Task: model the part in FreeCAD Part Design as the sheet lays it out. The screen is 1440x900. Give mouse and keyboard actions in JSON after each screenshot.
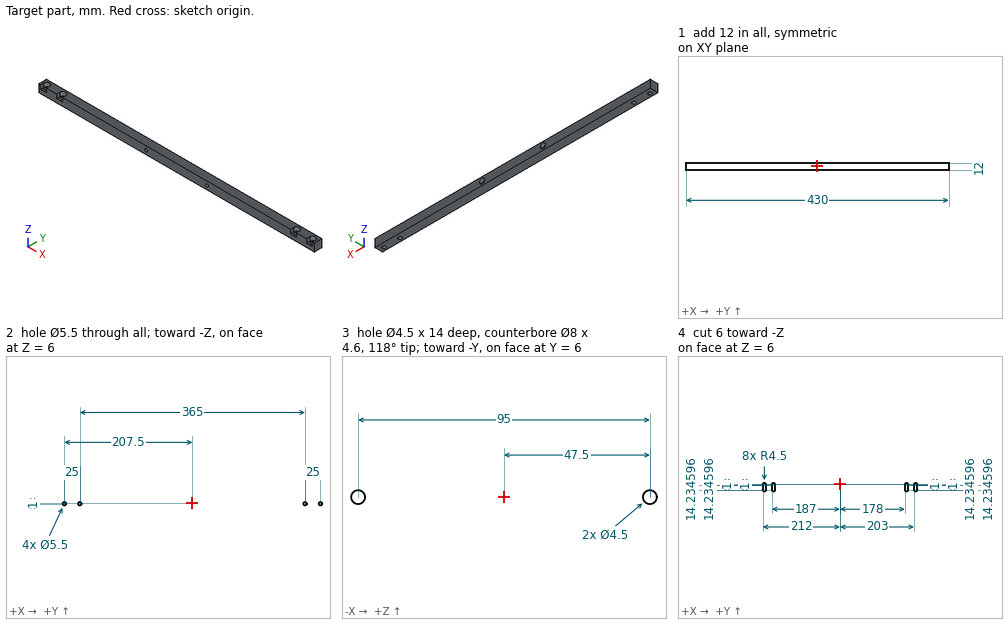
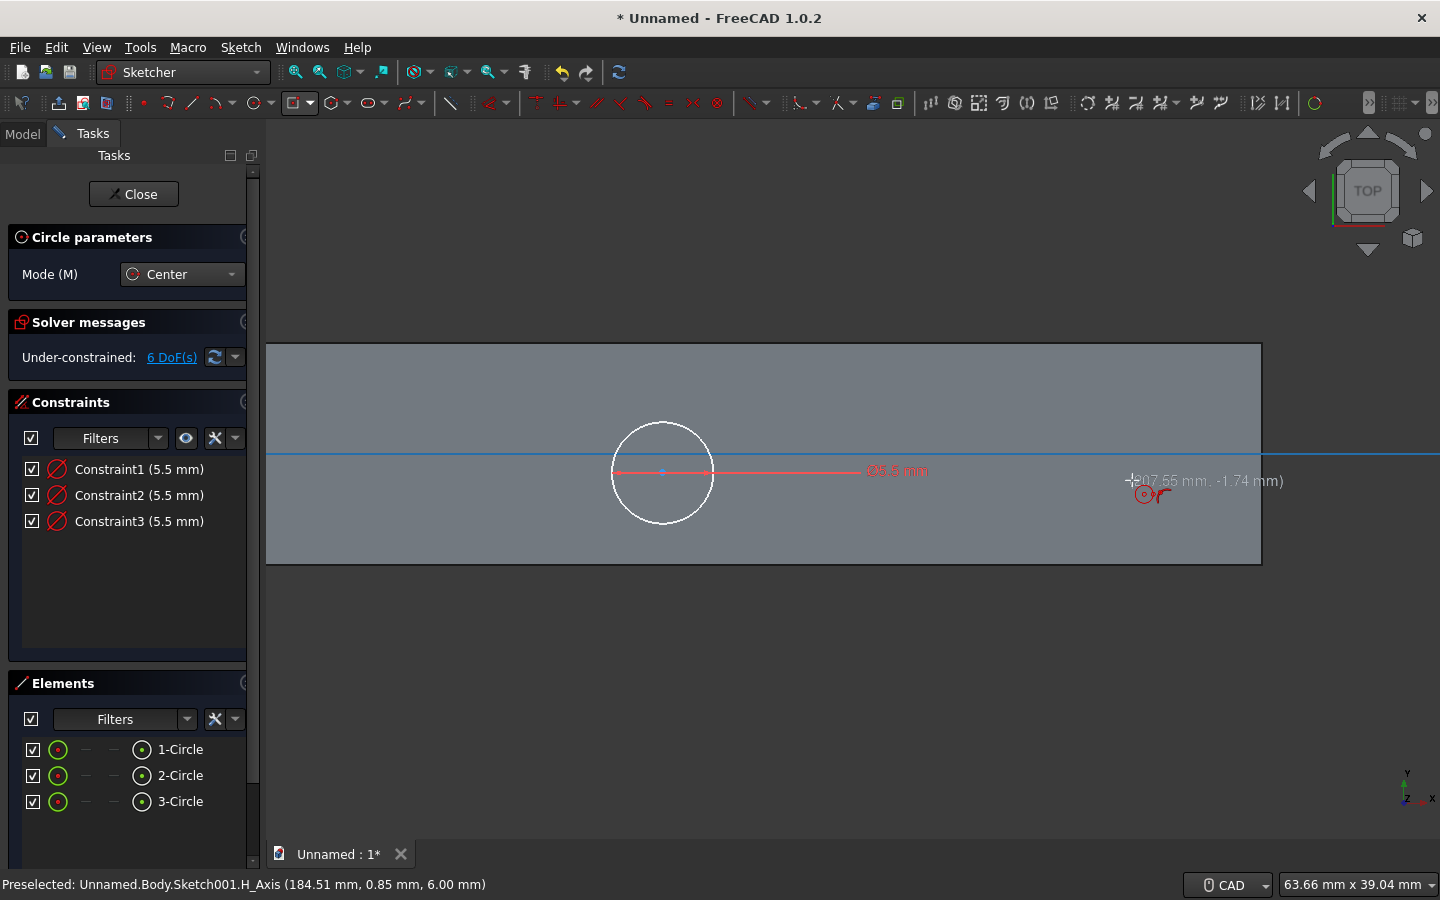
{"action": "left_click", "coordinate": [1124, 472]}
{"action": "mouse_move", "coordinate": [1160, 436]}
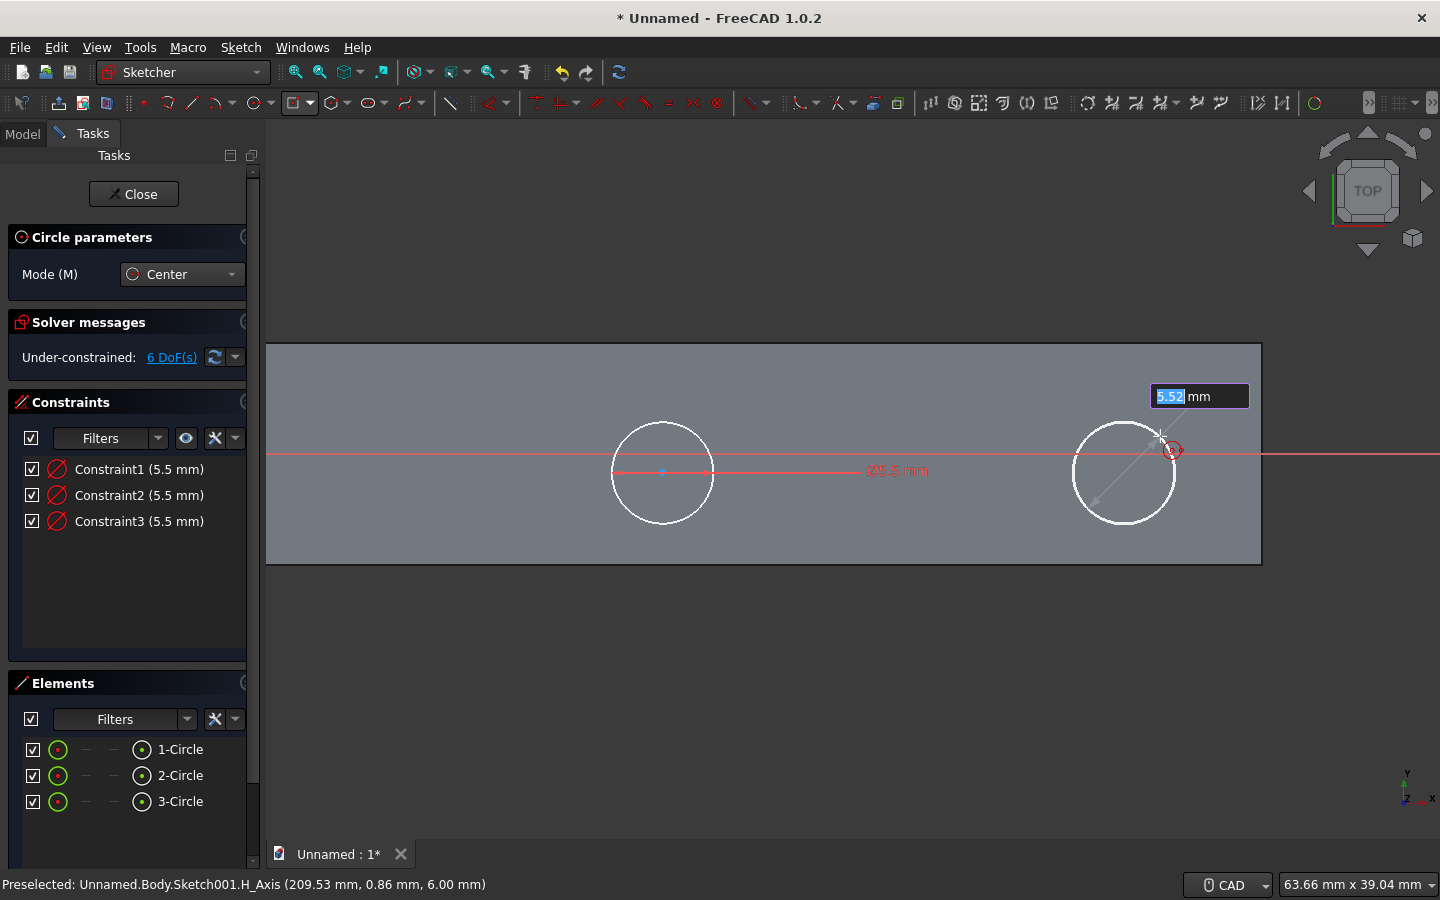
{"action": "type", "text": "5.5"}
{"action": "key", "text": "Return"}
{"action": "key", "text": "Escape"}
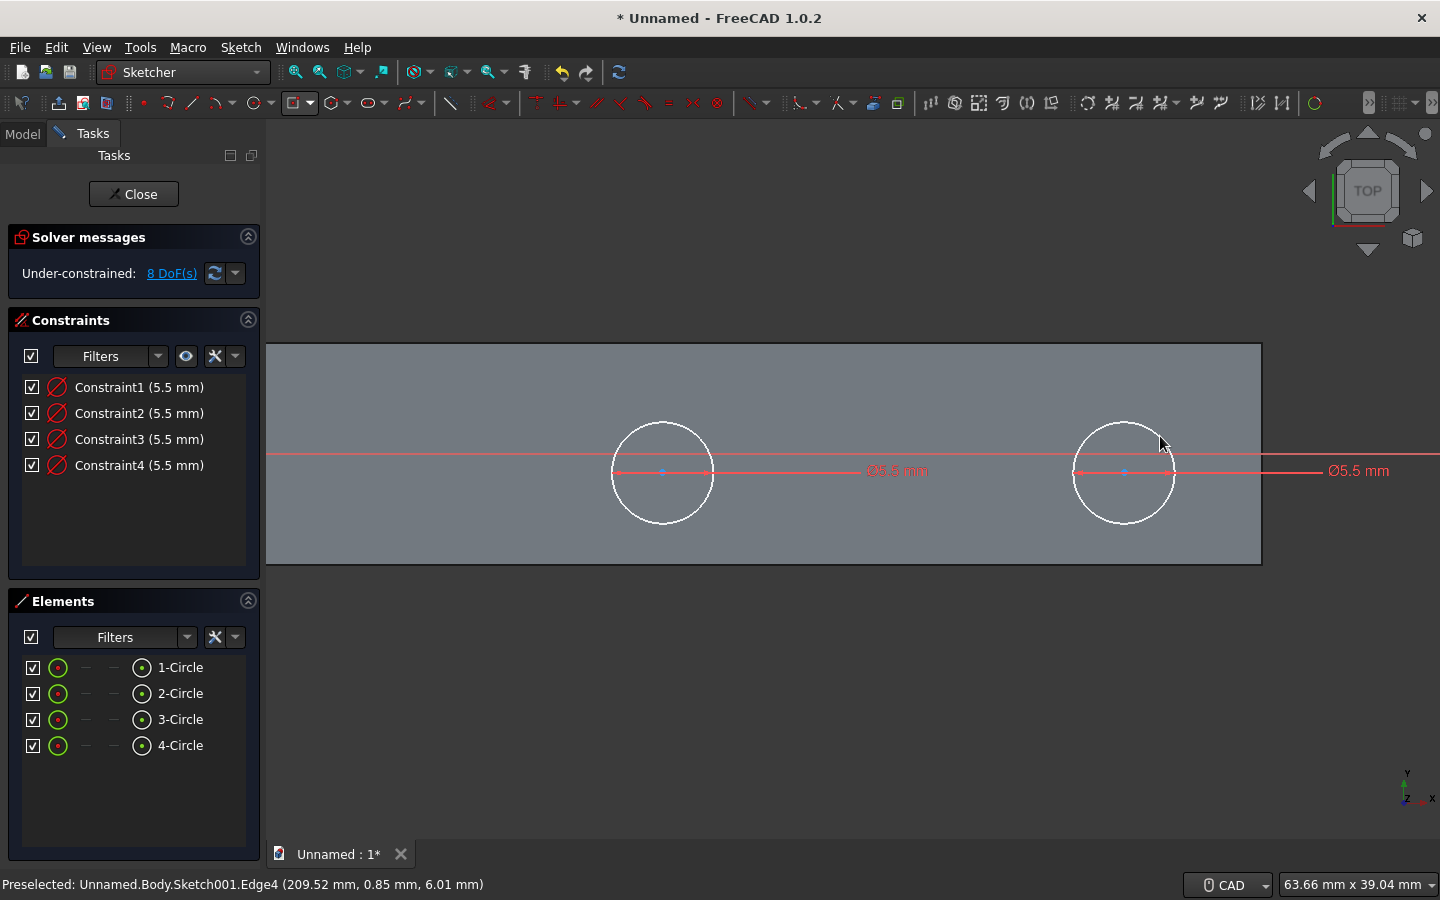
{"action": "scroll", "coordinate": [1132, 480], "scroll_direction": "down", "scroll_amount": 12}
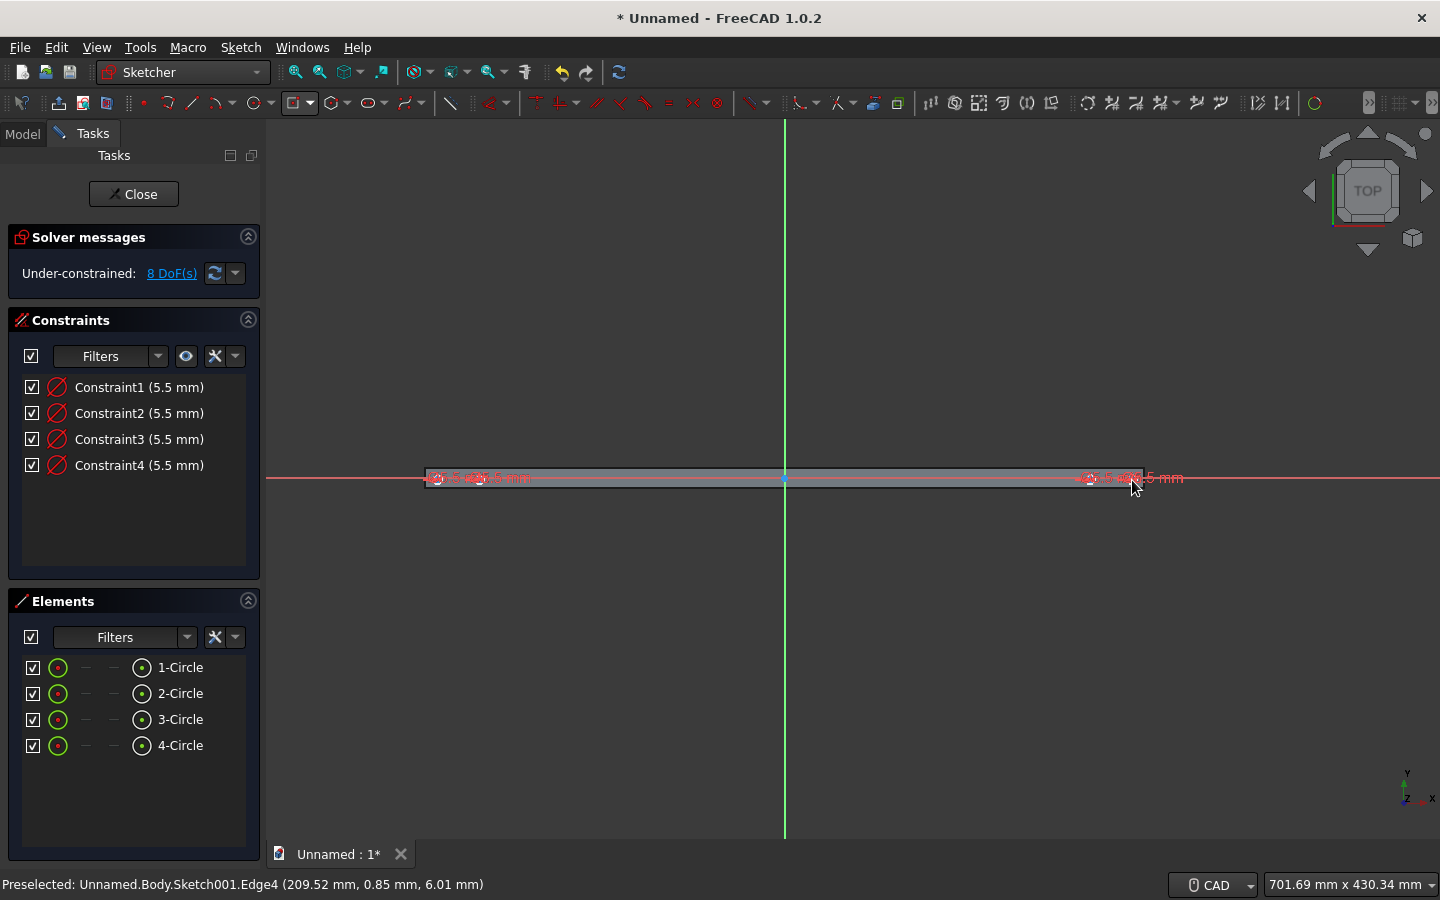
{"action": "left_click", "coordinate": [438, 480]}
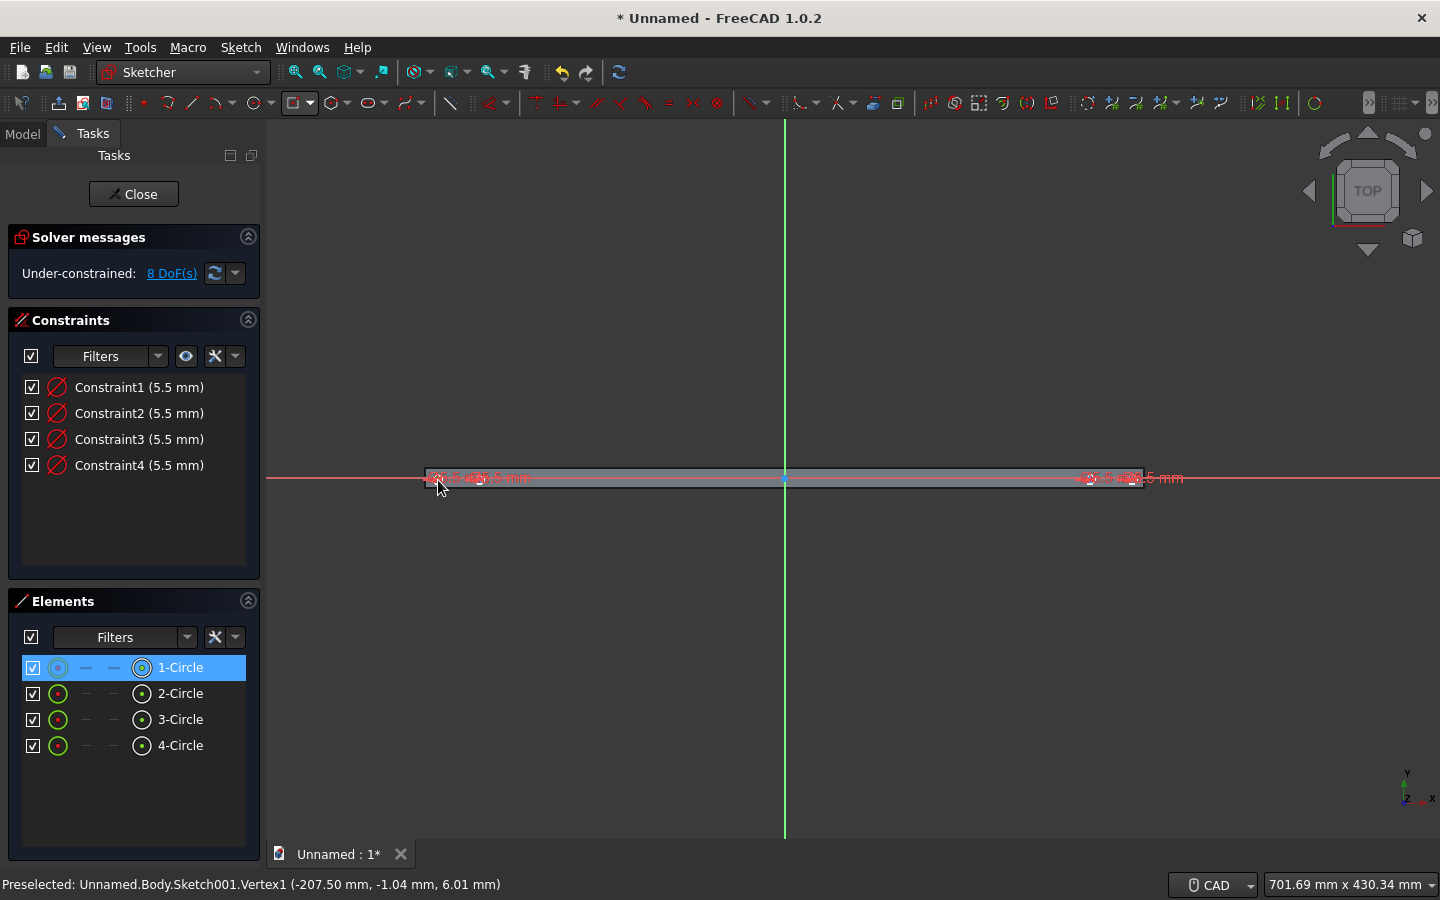
{"action": "left_click", "coordinate": [479, 480]}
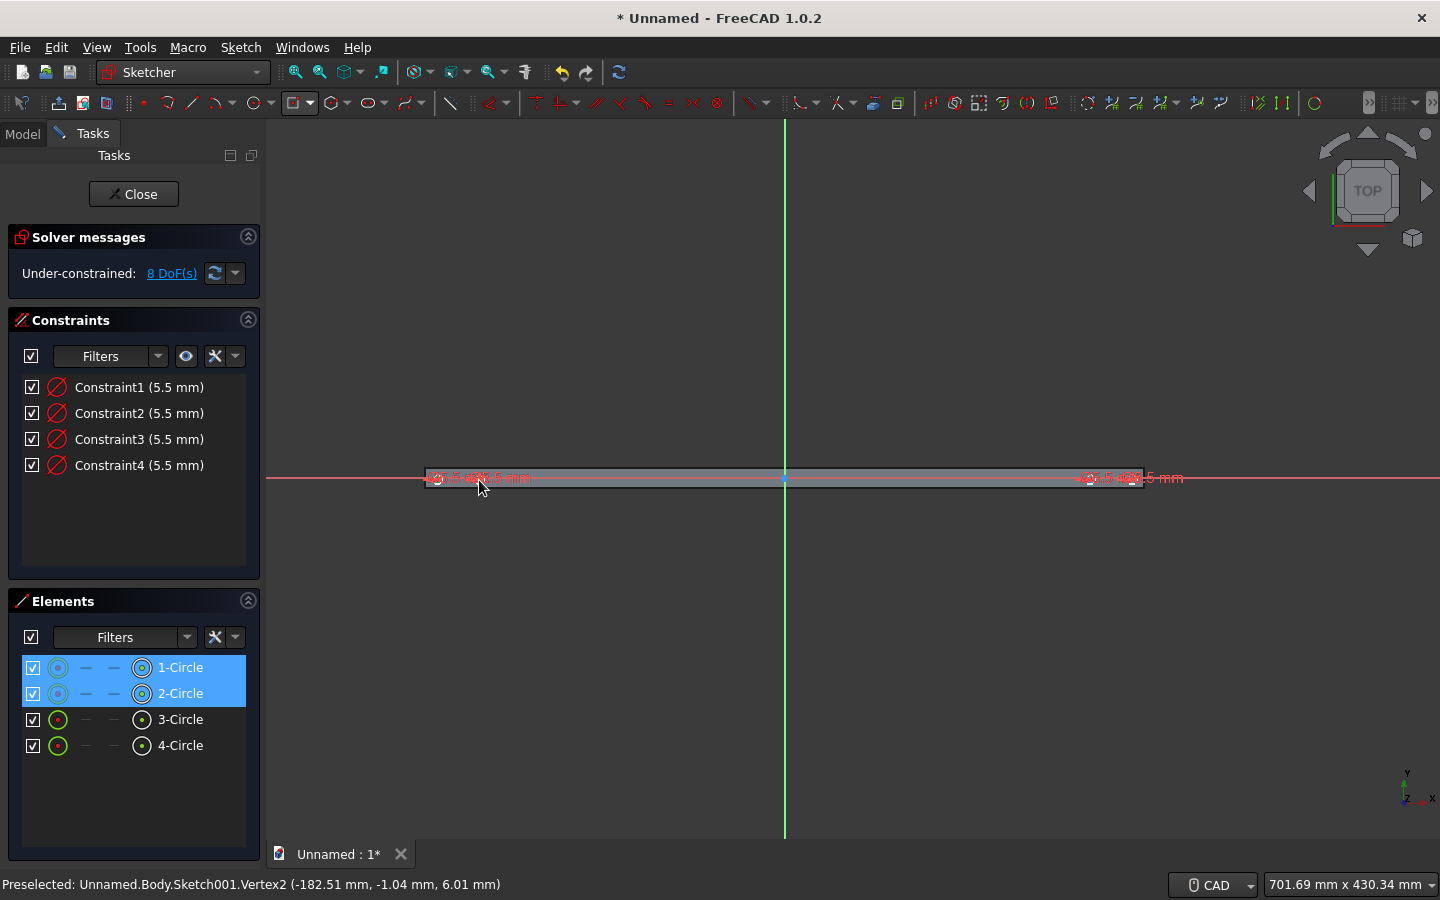
{"action": "left_click", "coordinate": [578, 104]}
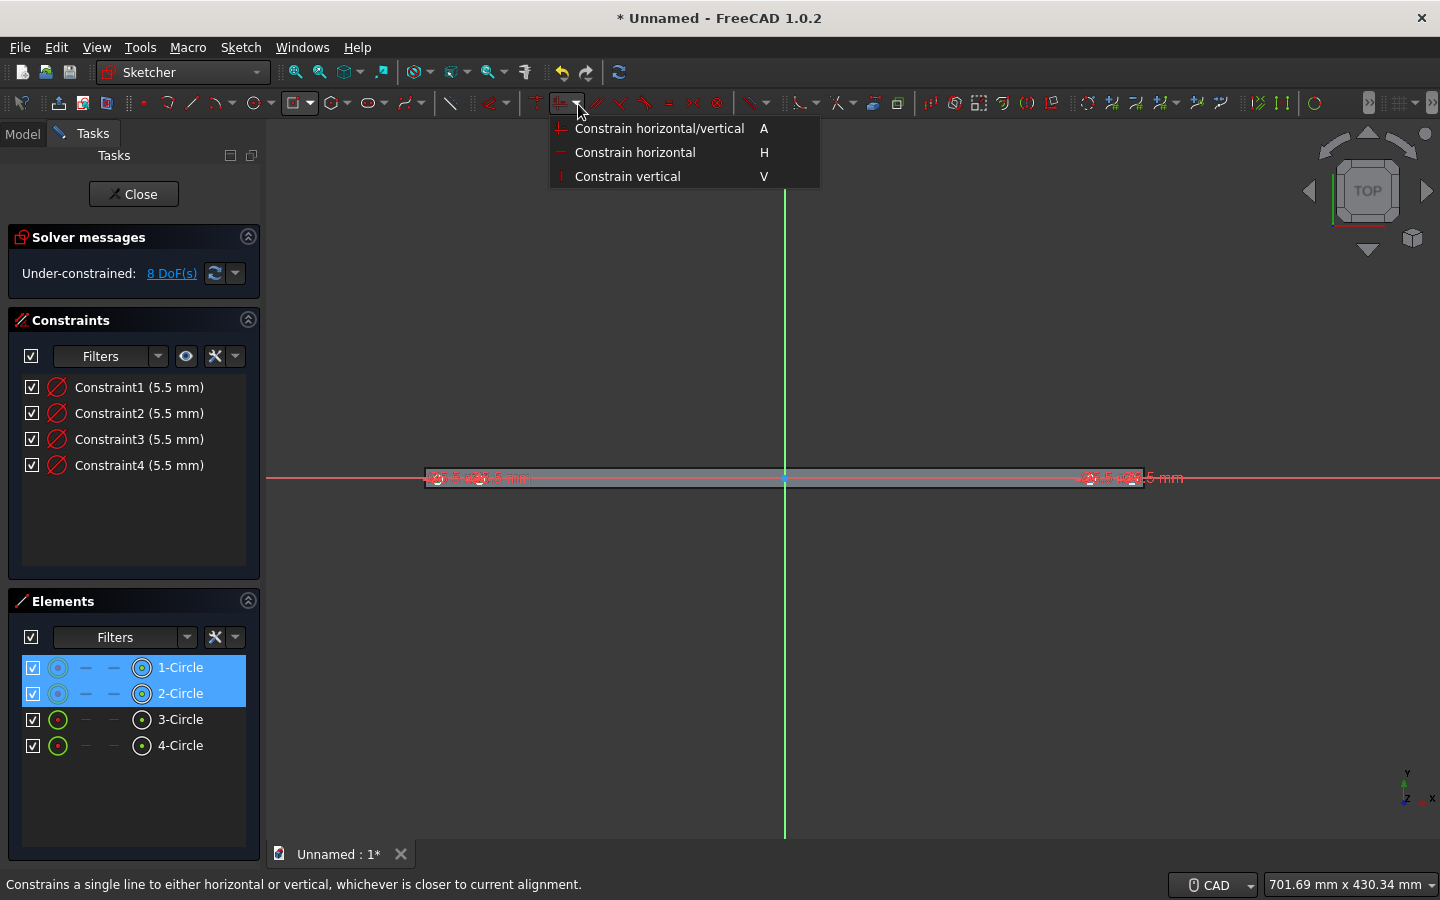
{"action": "left_click", "coordinate": [685, 152]}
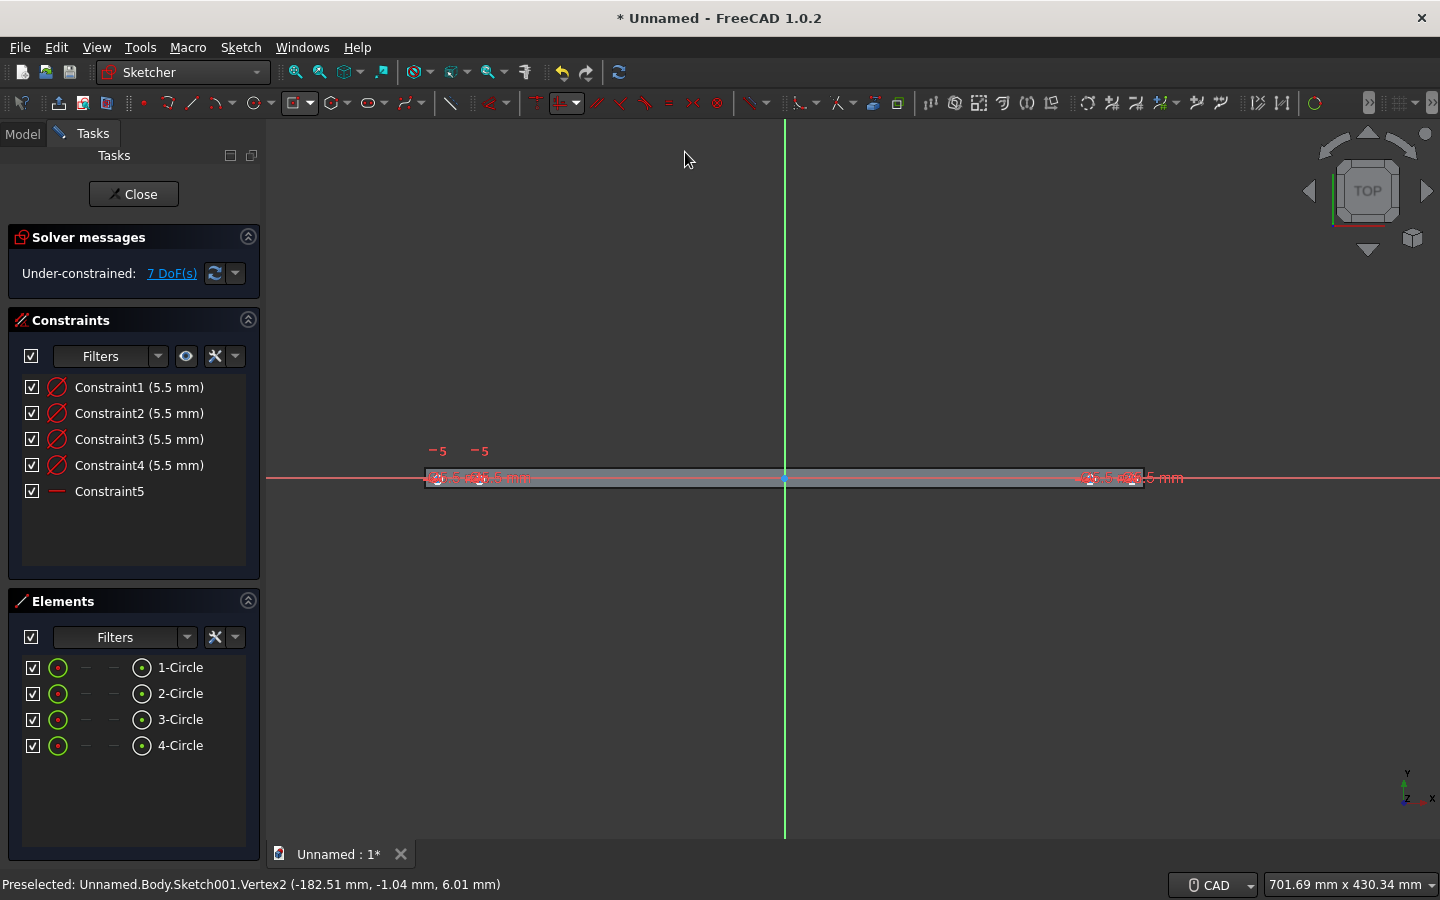
{"action": "left_click", "coordinate": [479, 480]}